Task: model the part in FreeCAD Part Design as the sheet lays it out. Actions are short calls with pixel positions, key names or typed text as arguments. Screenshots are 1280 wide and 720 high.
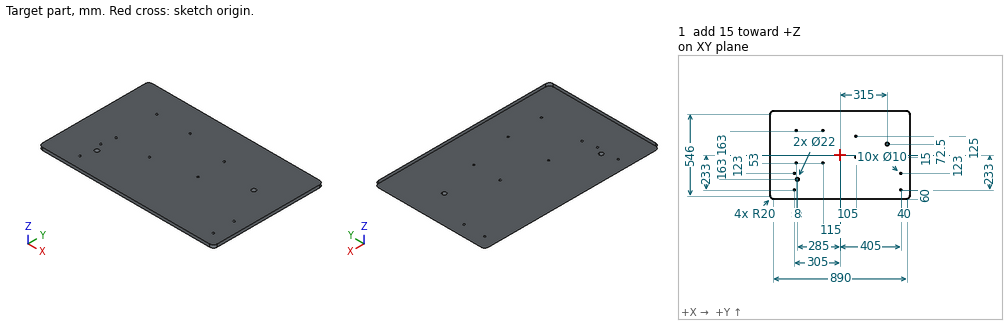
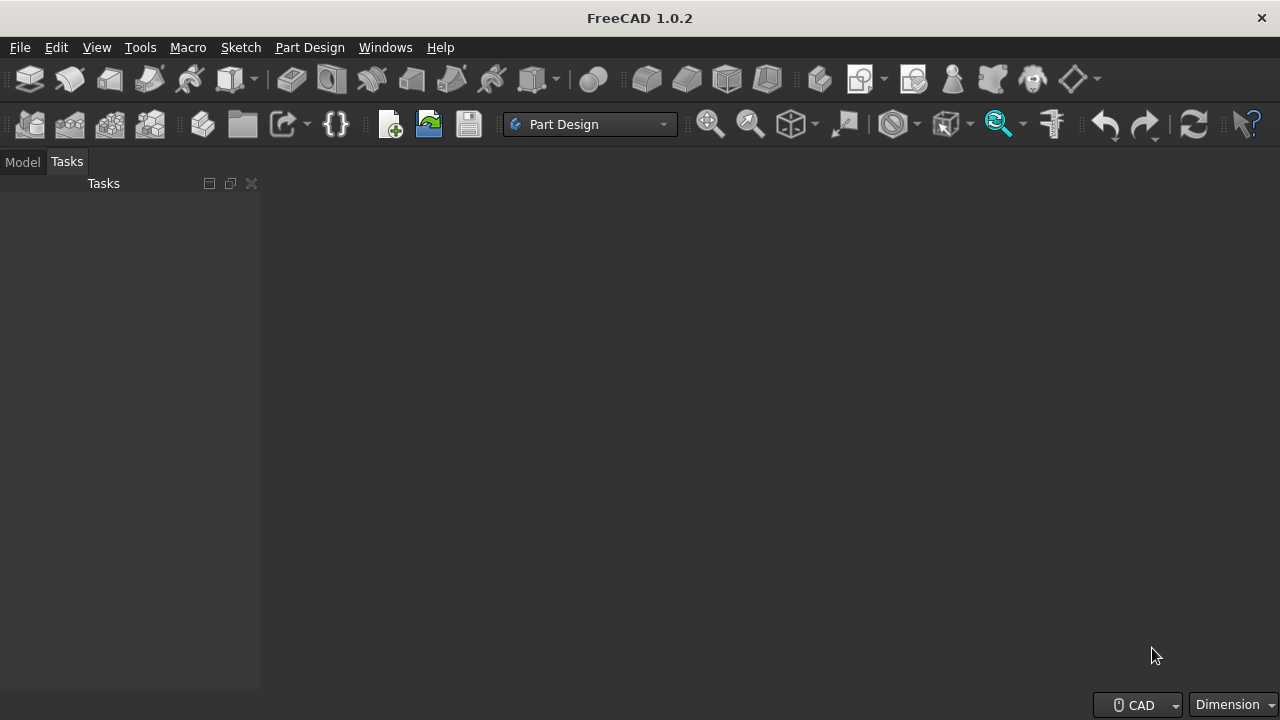
click(390, 124)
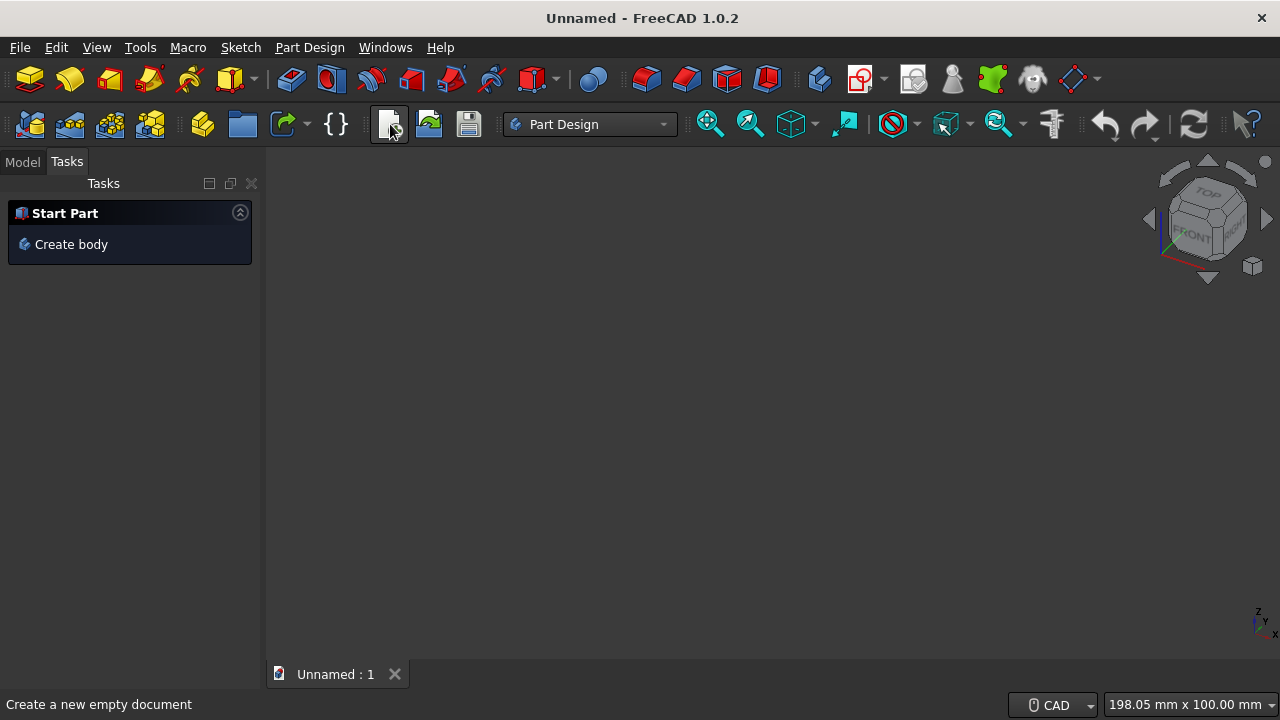
click(860, 80)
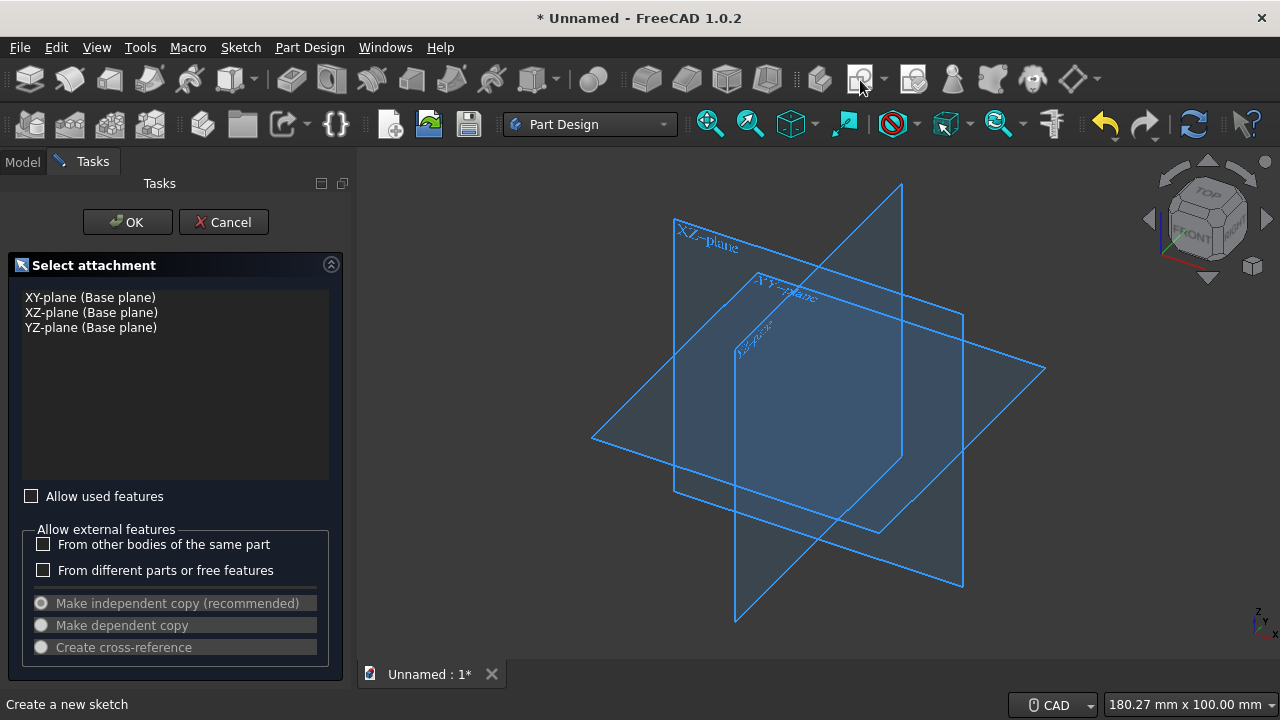
click(82, 298)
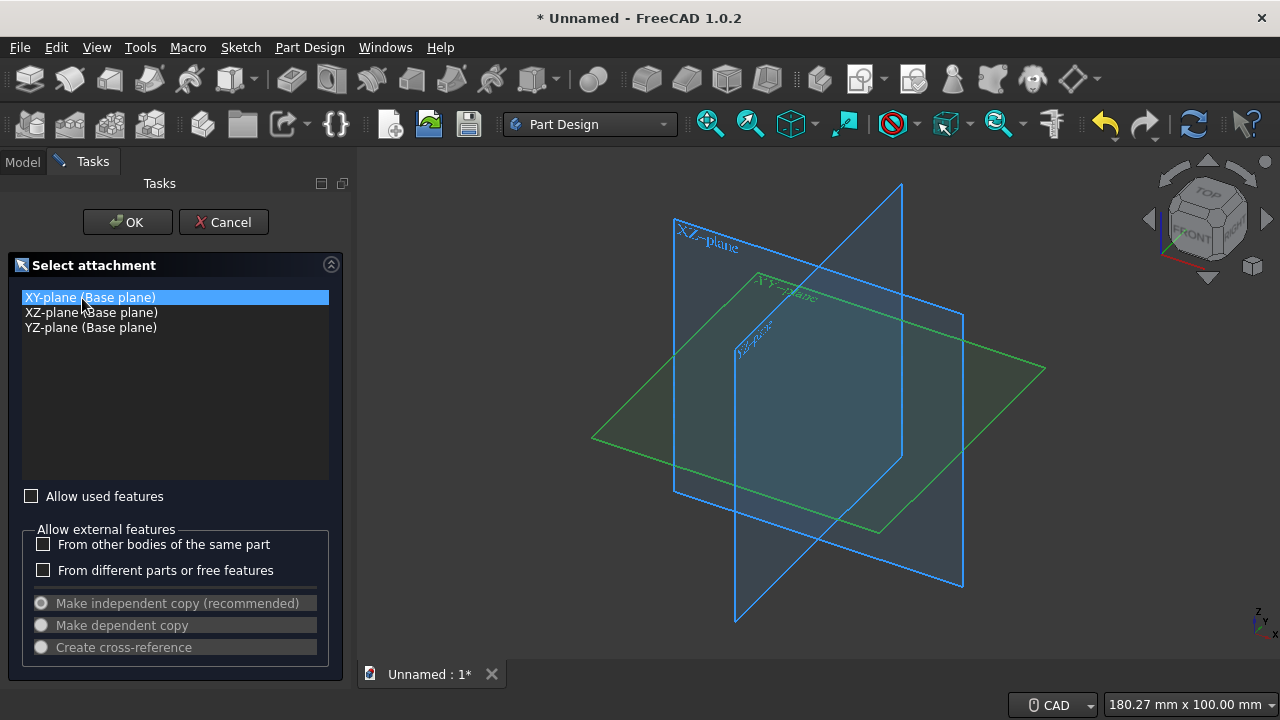
click(128, 222)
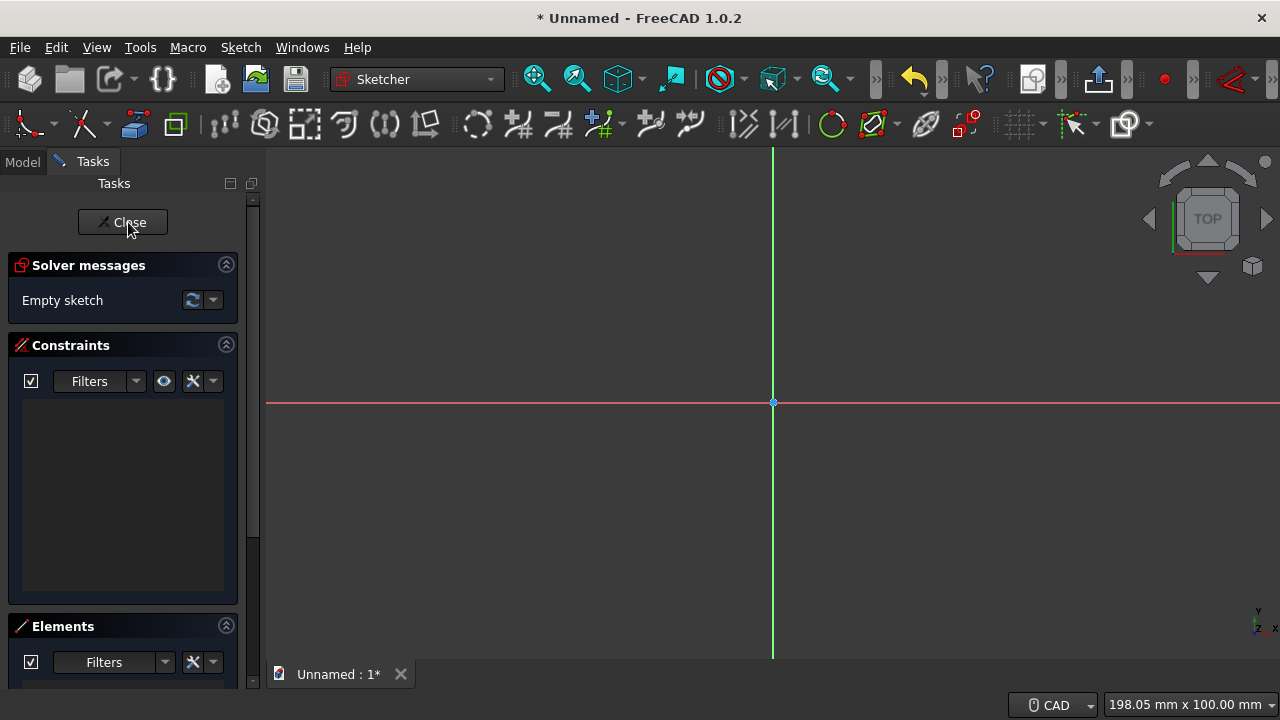
scroll(696, 403, down, 11)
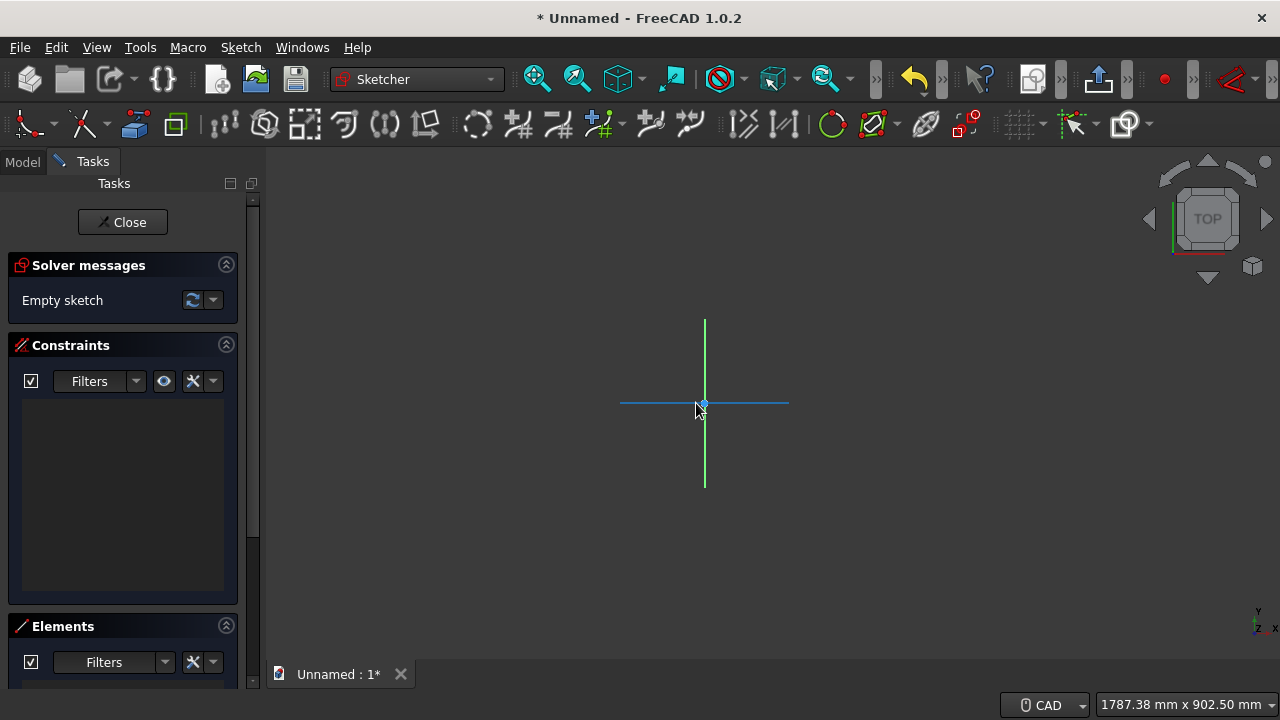
key(g)
key(l)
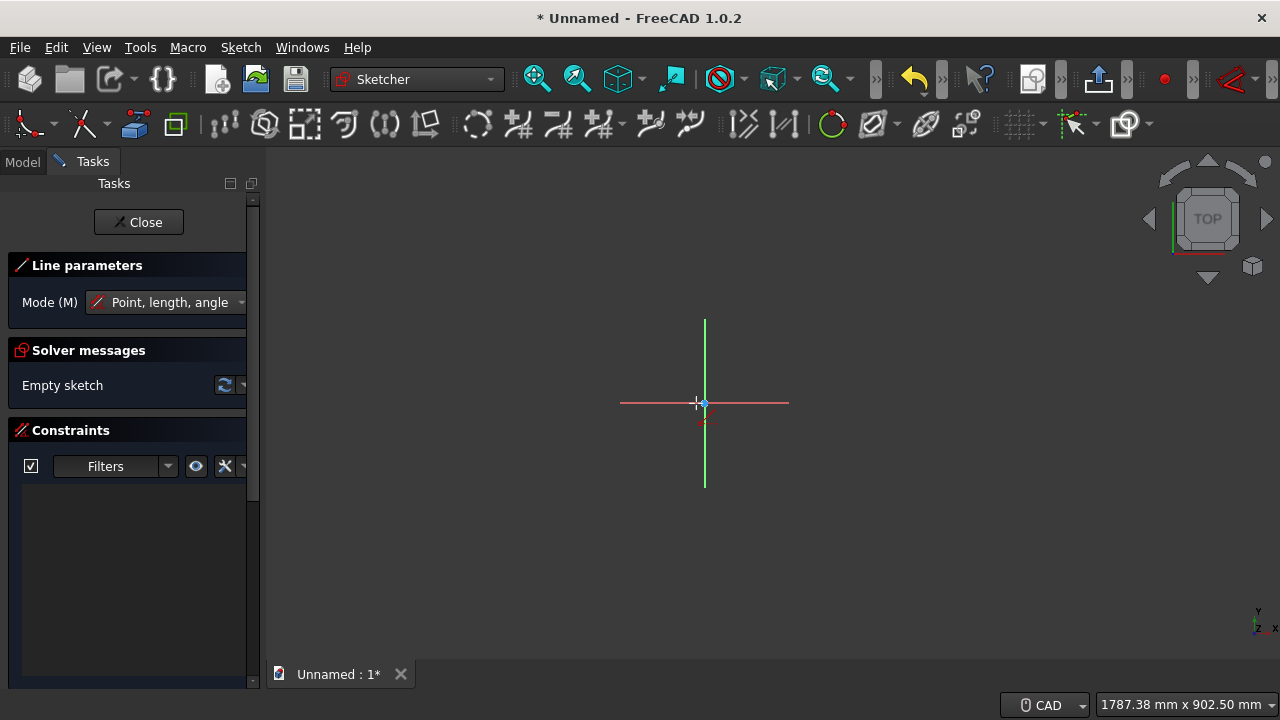
click(441, 249)
click(441, 558)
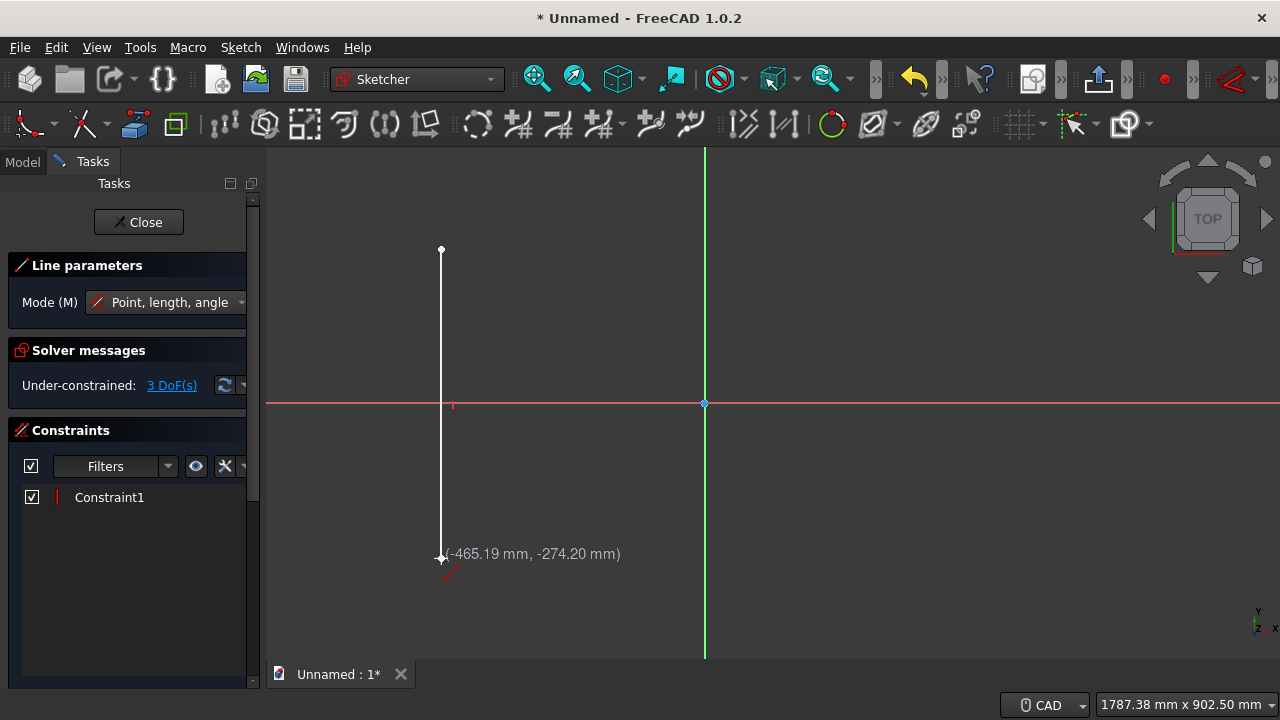
click(452, 570)
click(957, 570)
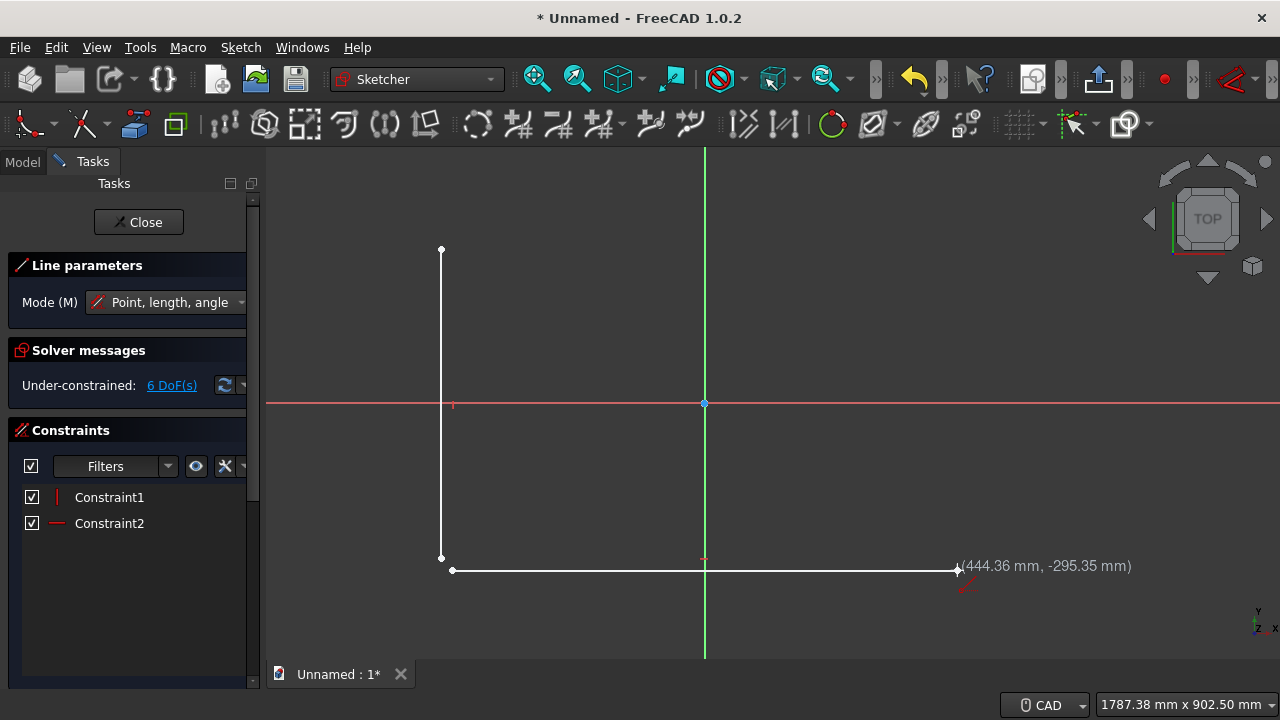
click(969, 558)
click(969, 249)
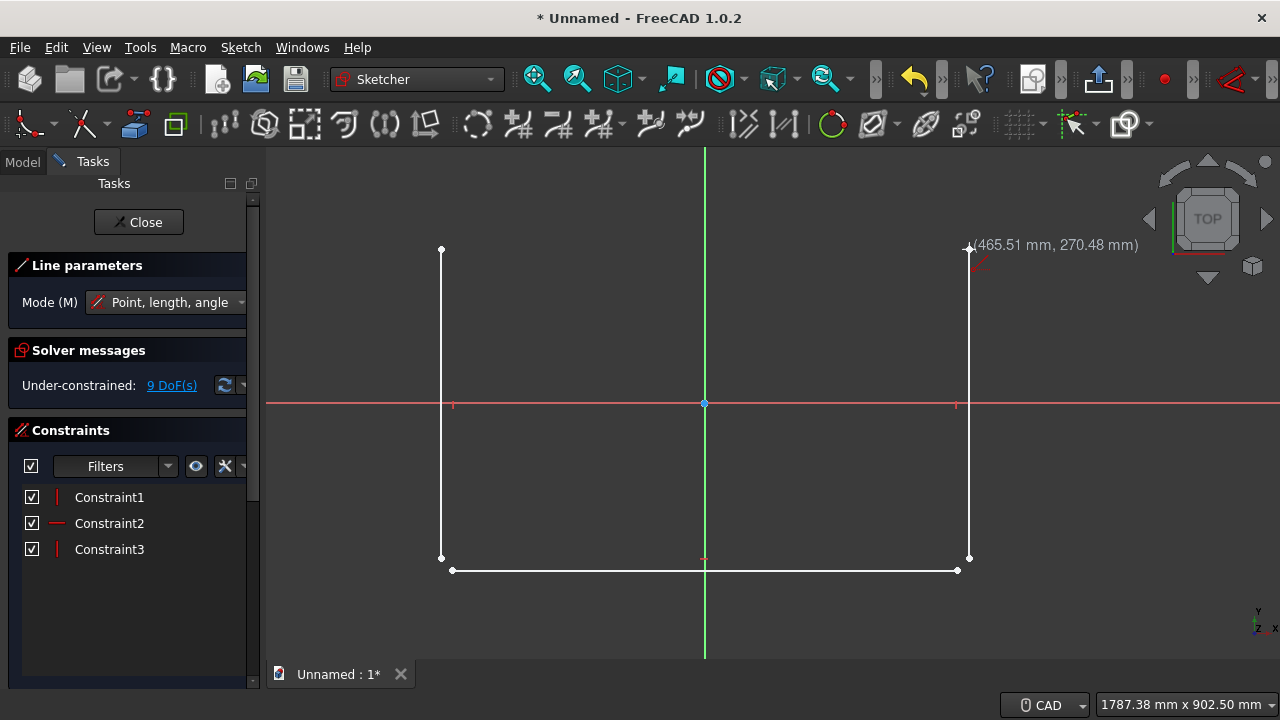
click(957, 237)
click(452, 237)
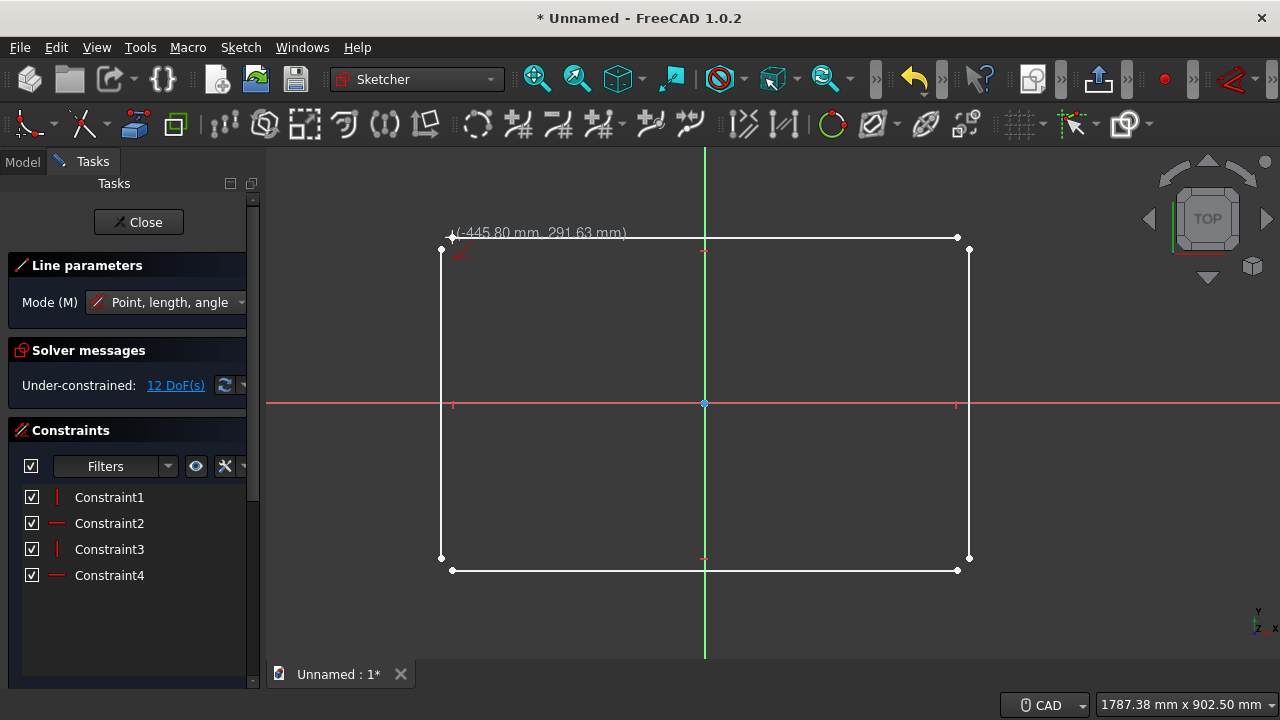
key(g)
key(3)
key(a)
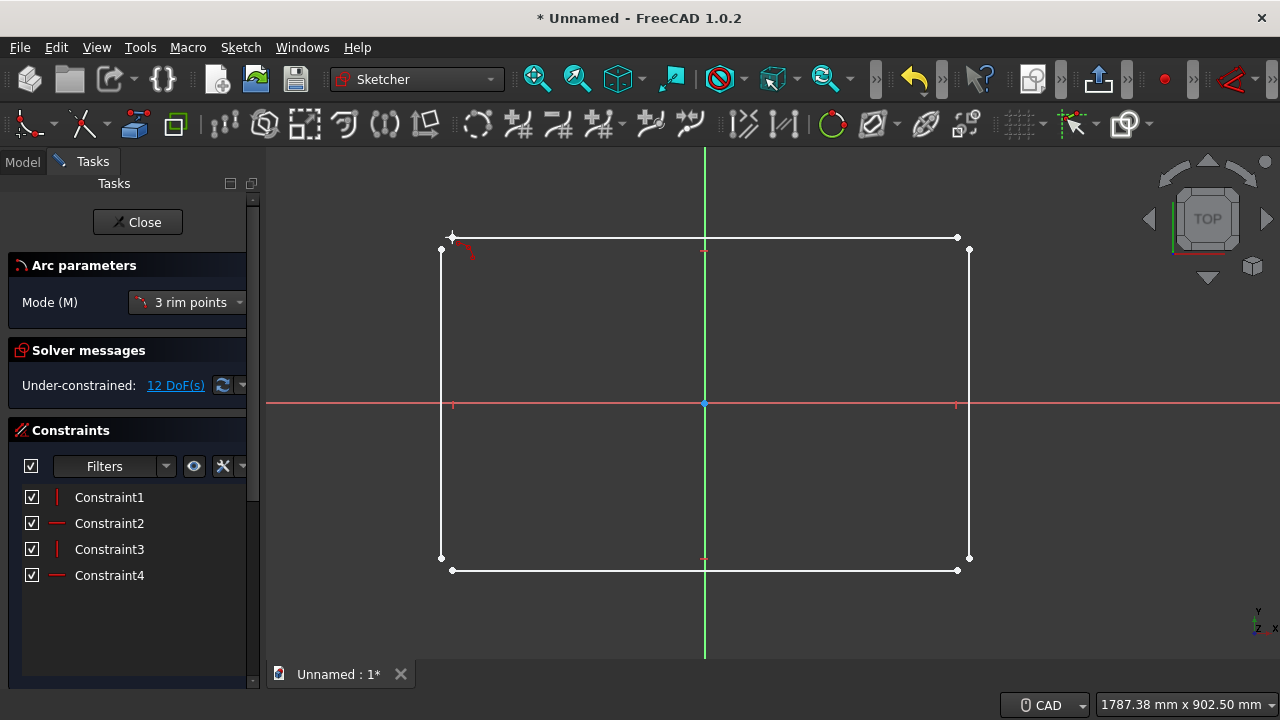
click(441, 559)
click(452, 571)